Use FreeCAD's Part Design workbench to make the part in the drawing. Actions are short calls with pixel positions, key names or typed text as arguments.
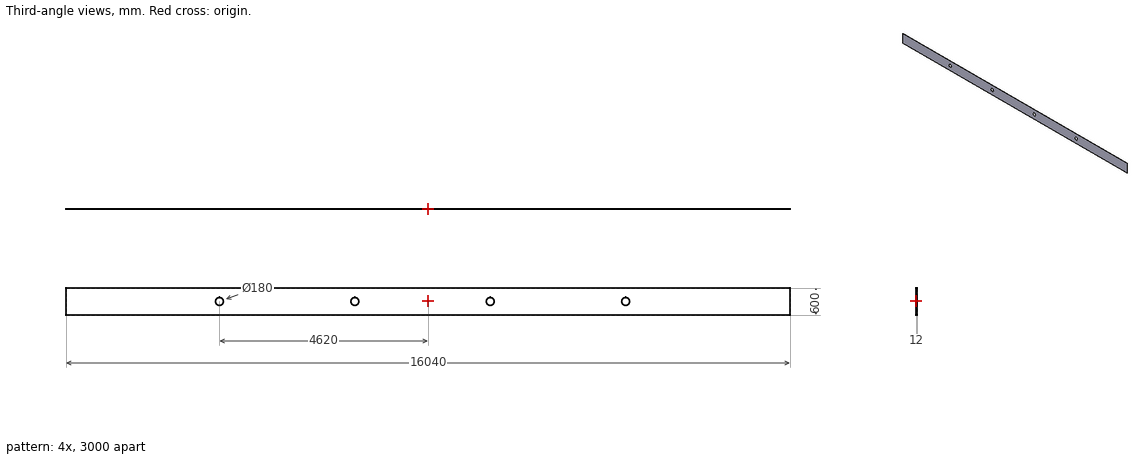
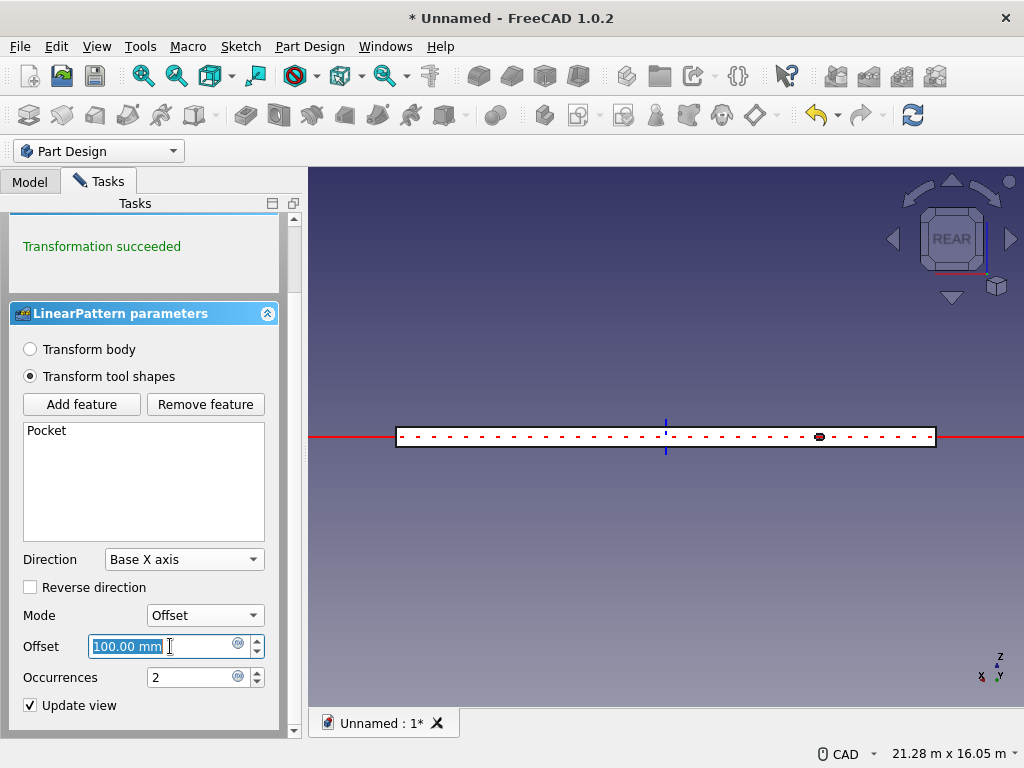
text(3000)
key(Tab)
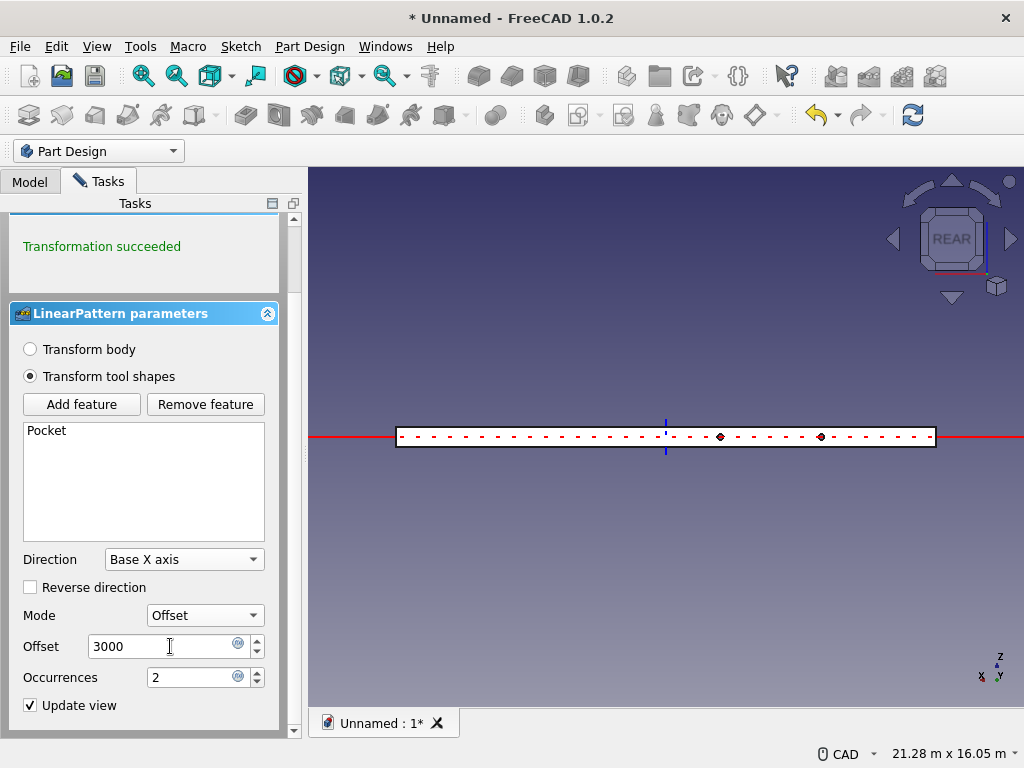
triple_click(199, 678)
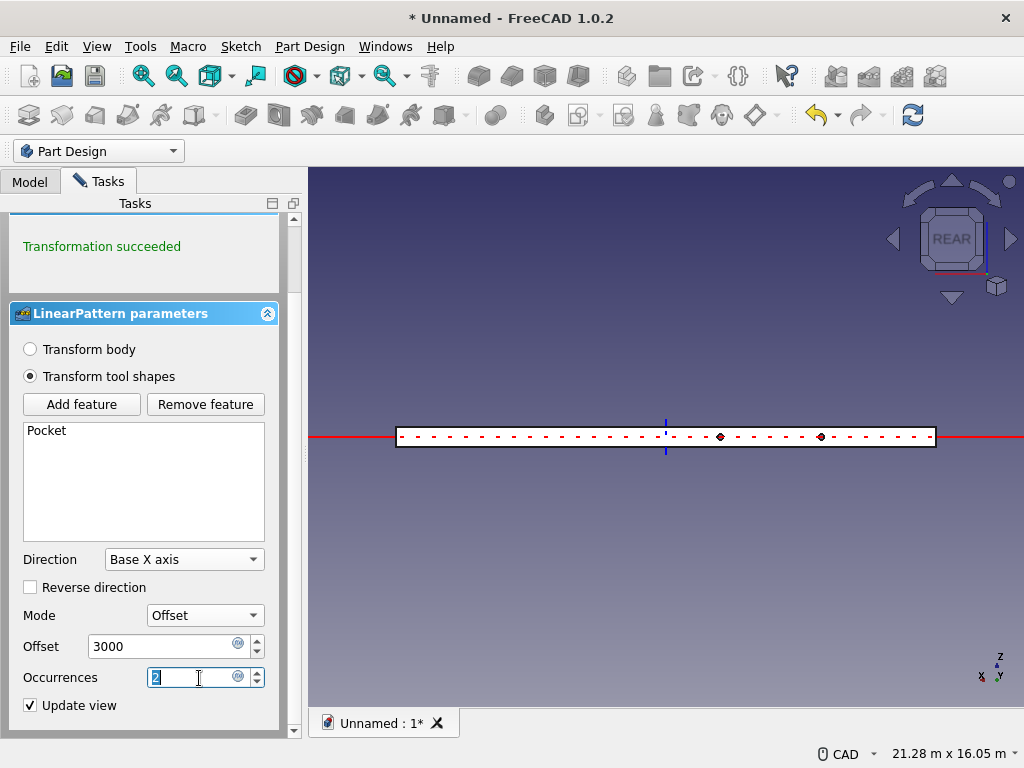
text(4)
key(Tab)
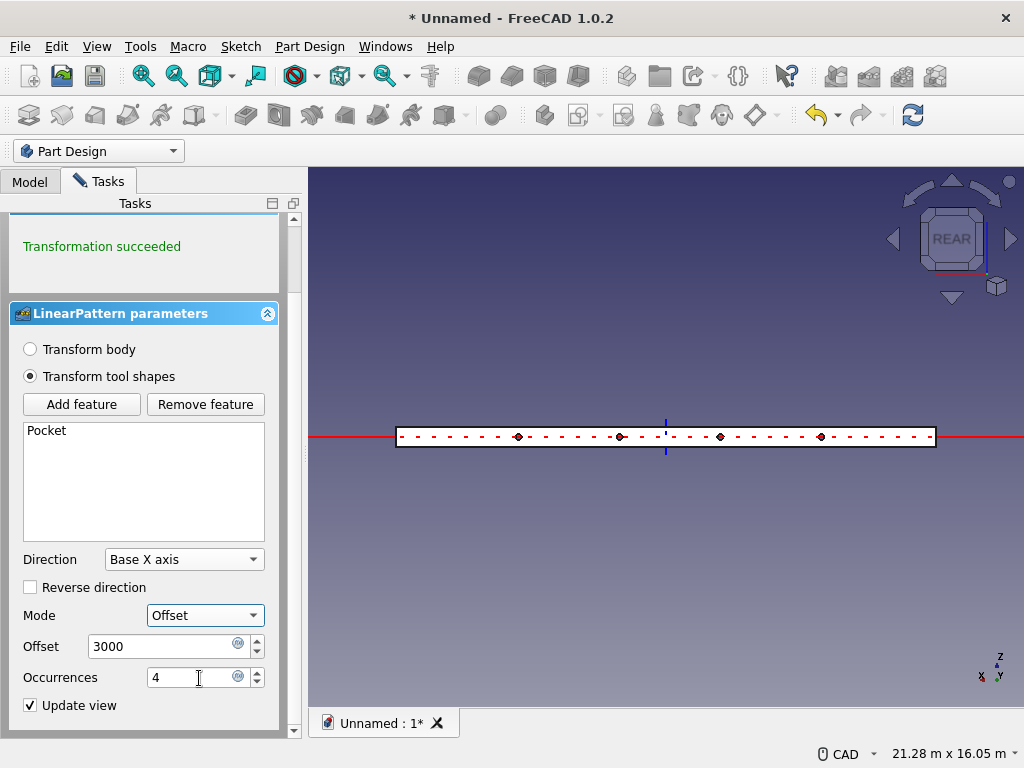
scroll(294, 476, up, 3)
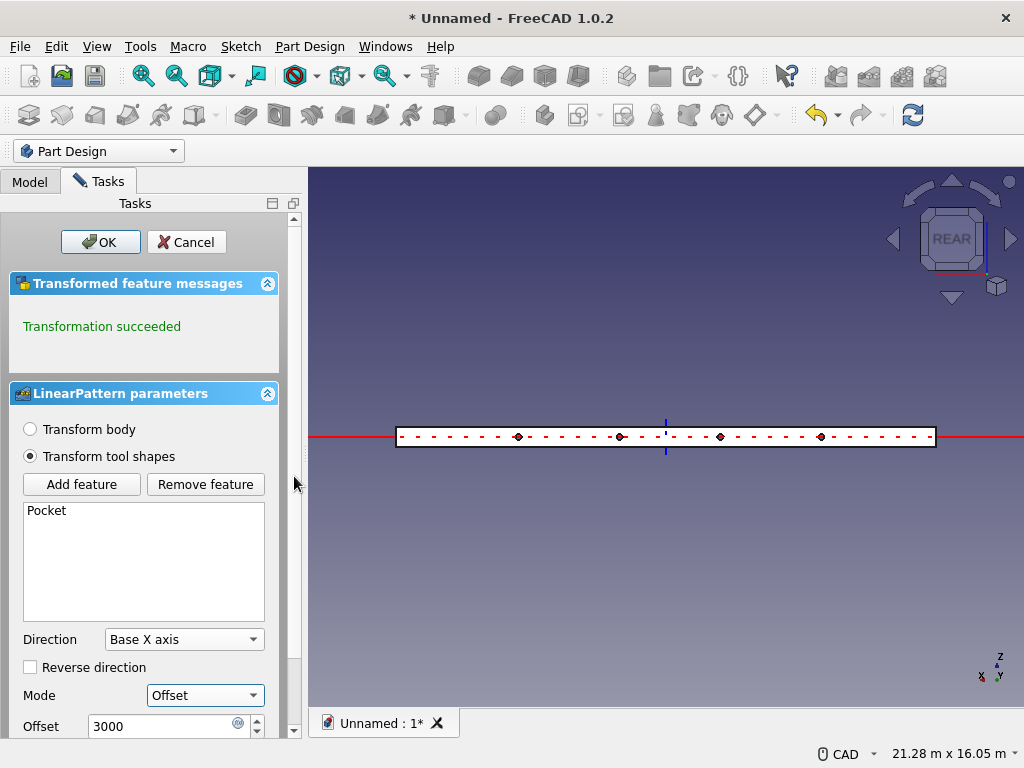
click(101, 242)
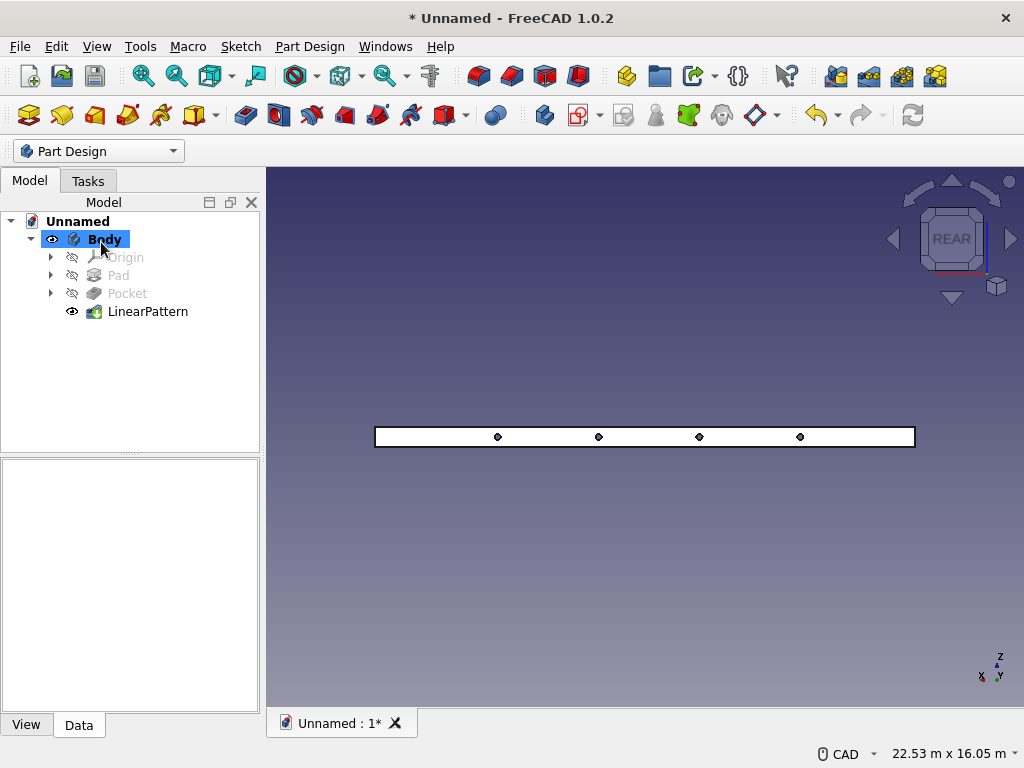
key(0)